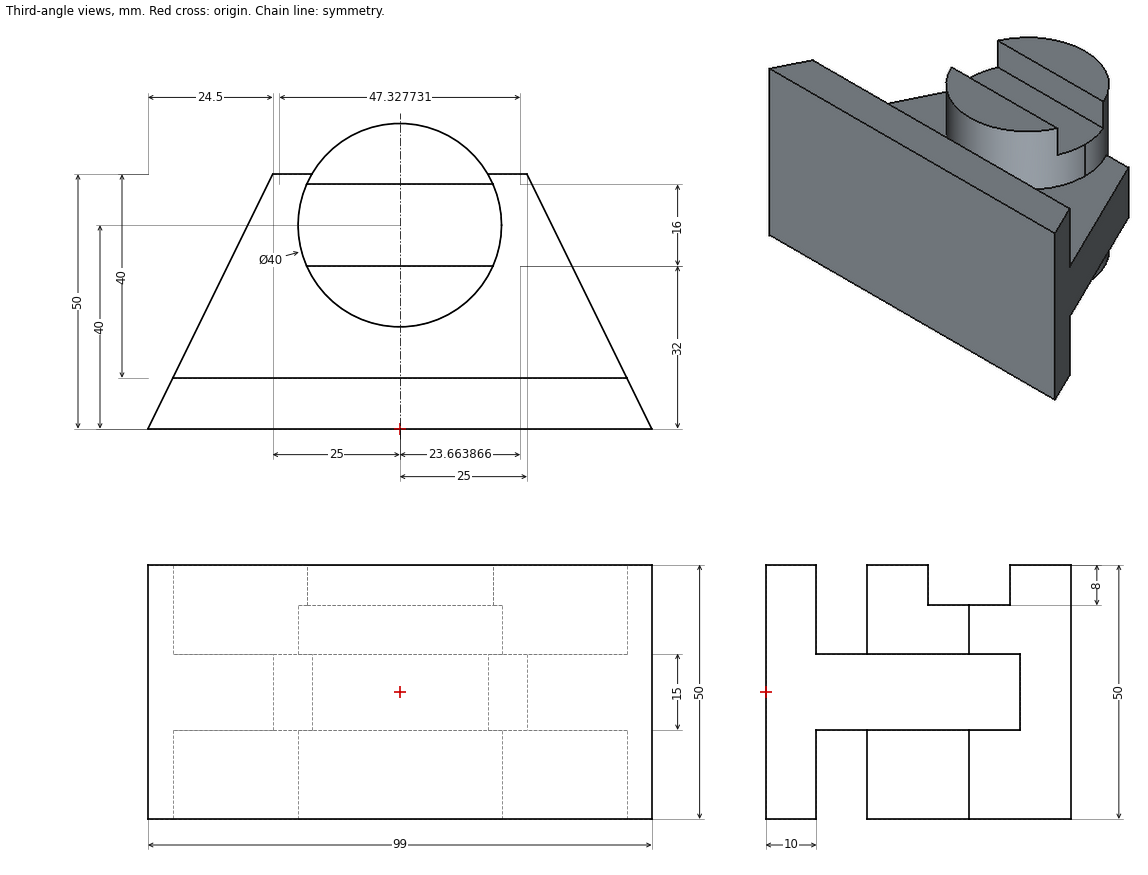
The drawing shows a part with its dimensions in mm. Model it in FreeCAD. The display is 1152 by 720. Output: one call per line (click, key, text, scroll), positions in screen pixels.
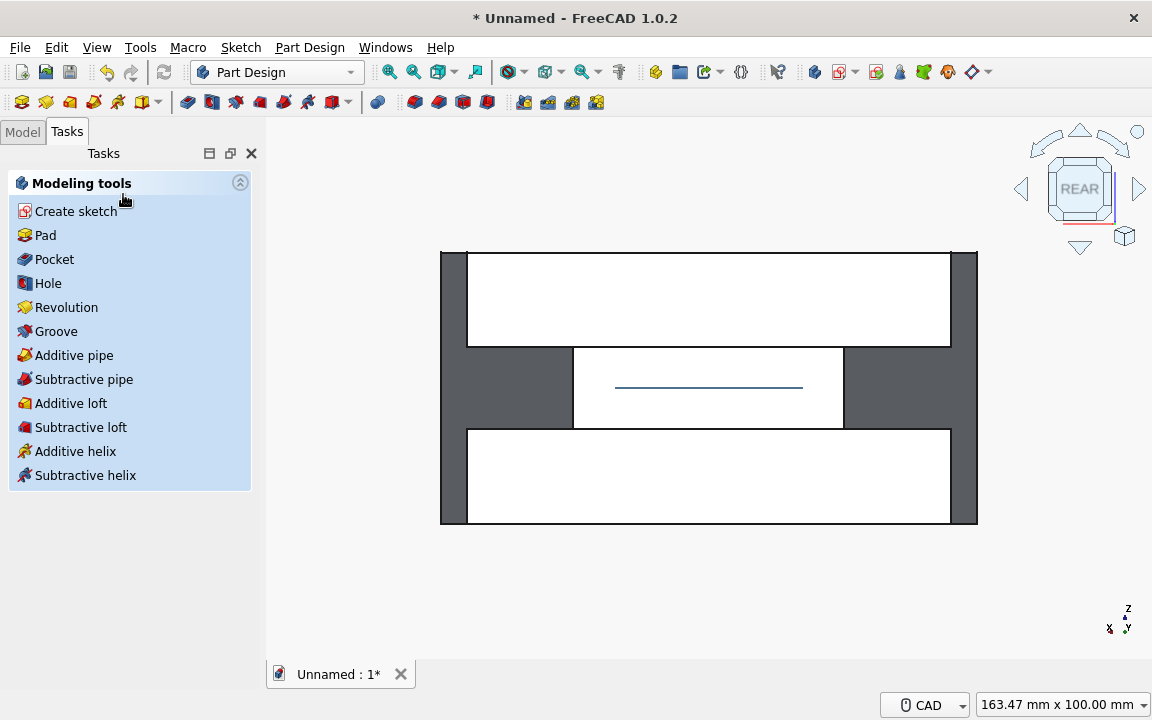
click(22, 102)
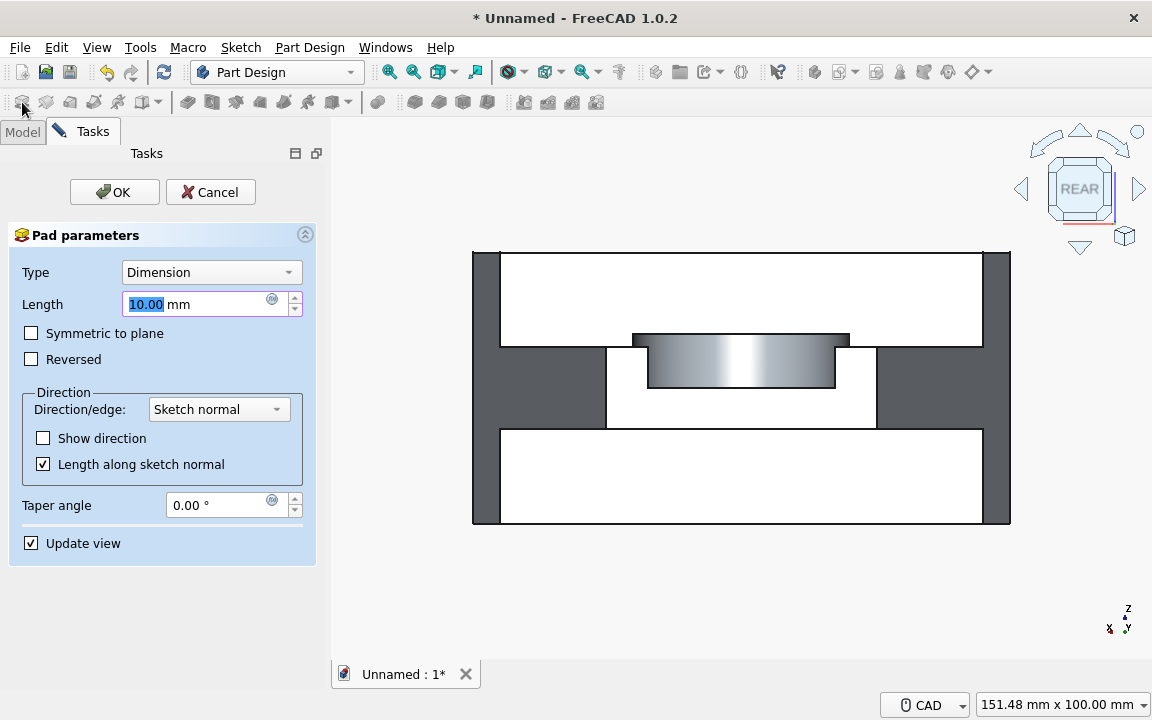
text(50)
key(Tab)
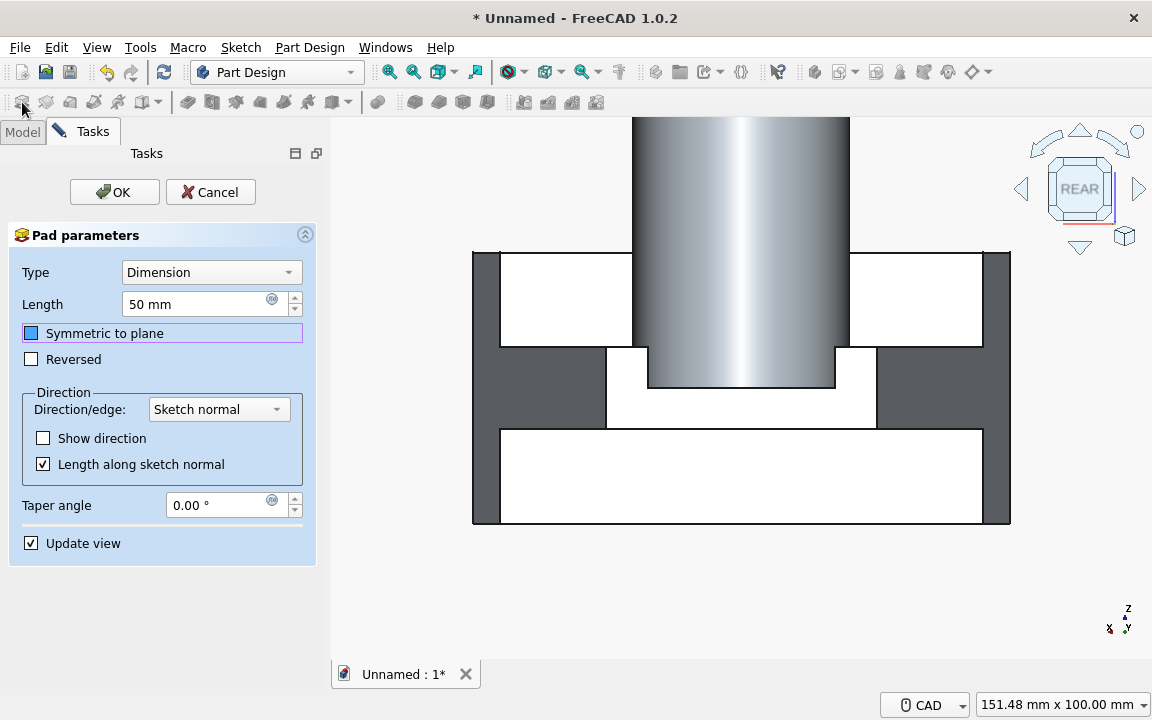
click(30, 333)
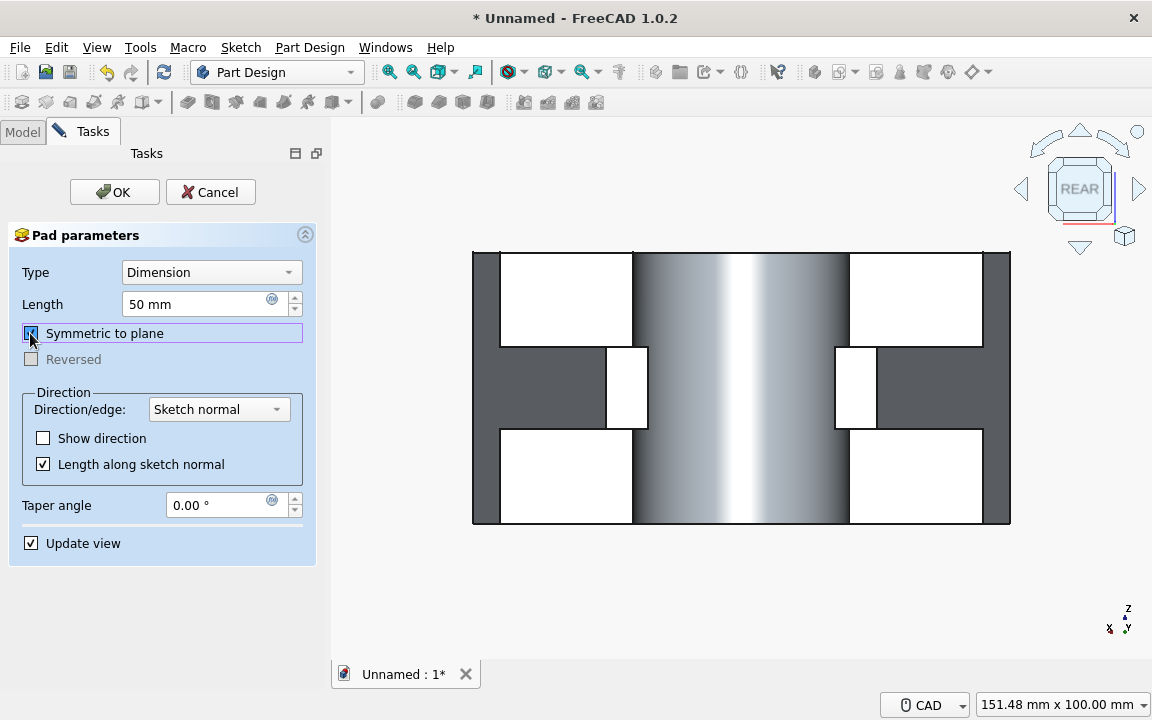
click(115, 192)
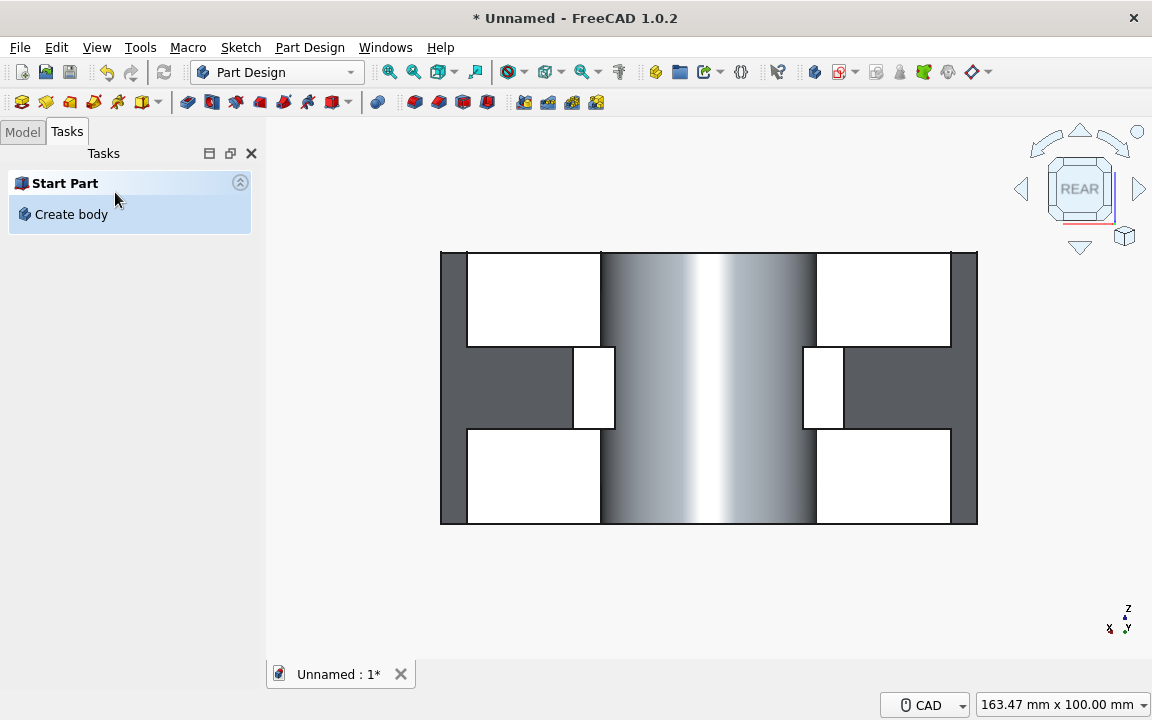
key(0)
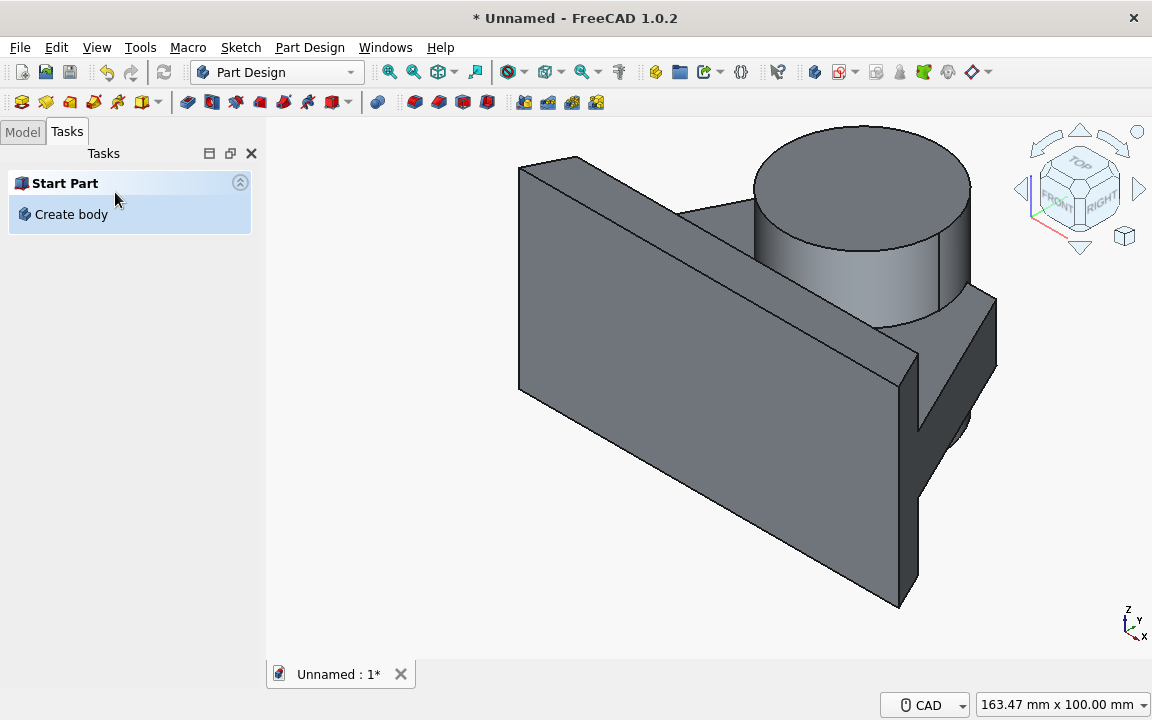
key(v)
key(f)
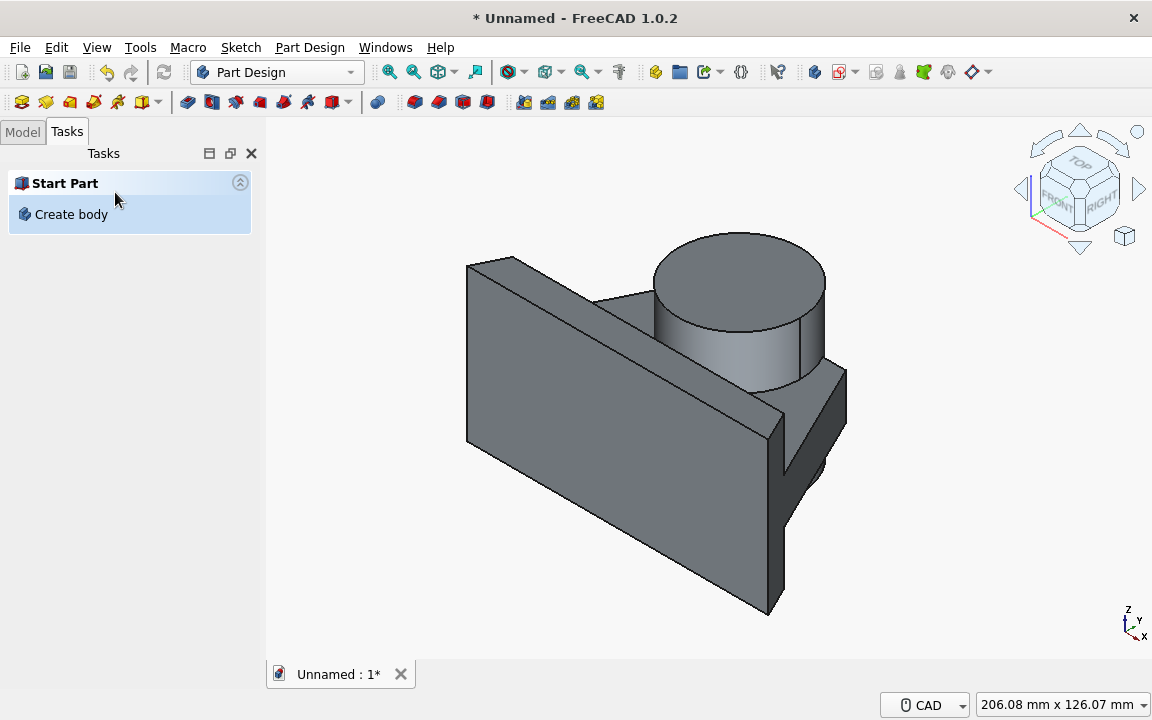
click(740, 282)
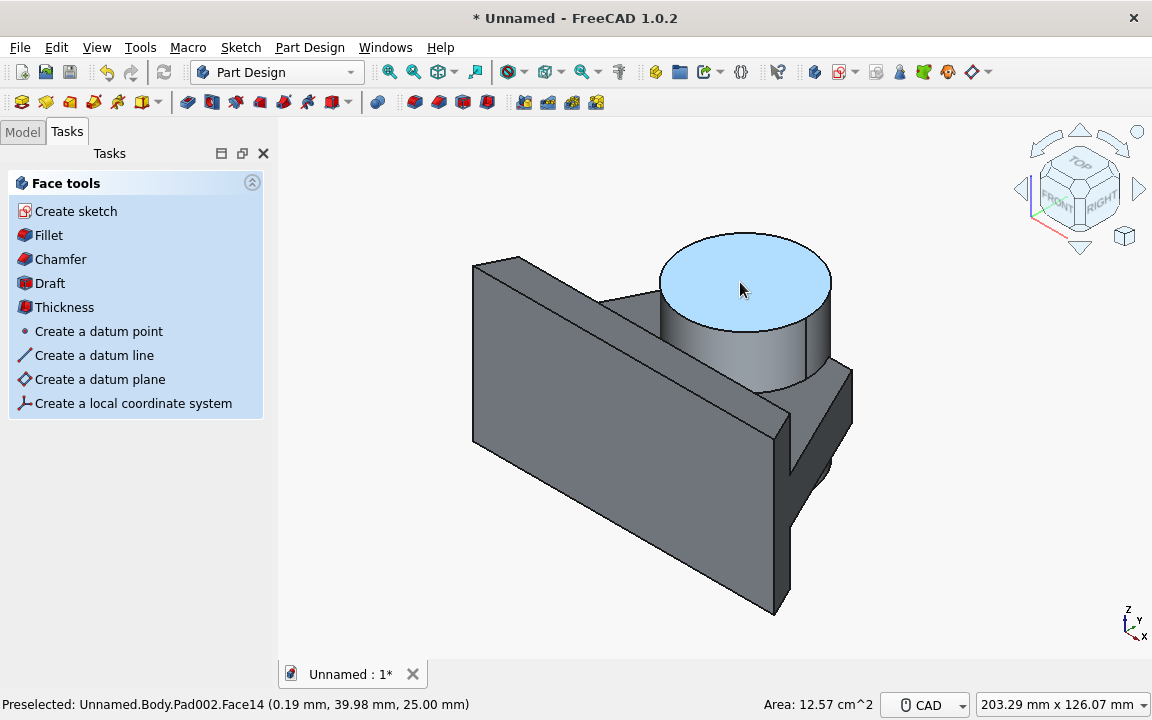
click(840, 72)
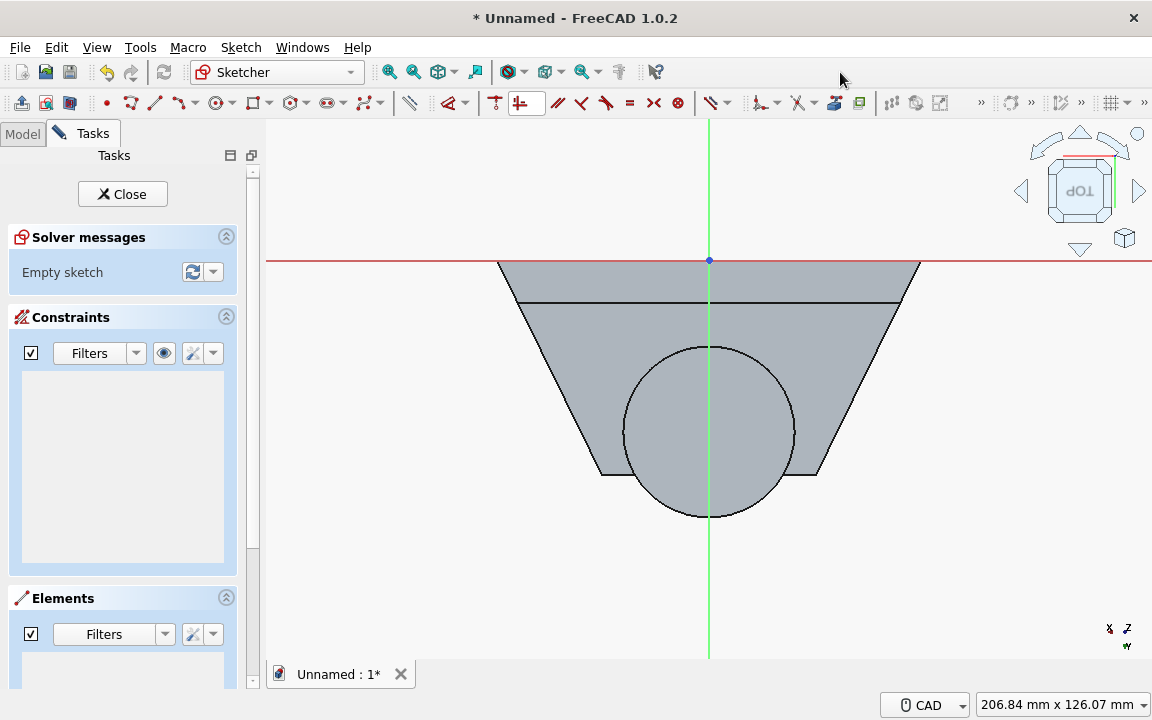
scroll(792, 332, up, 3)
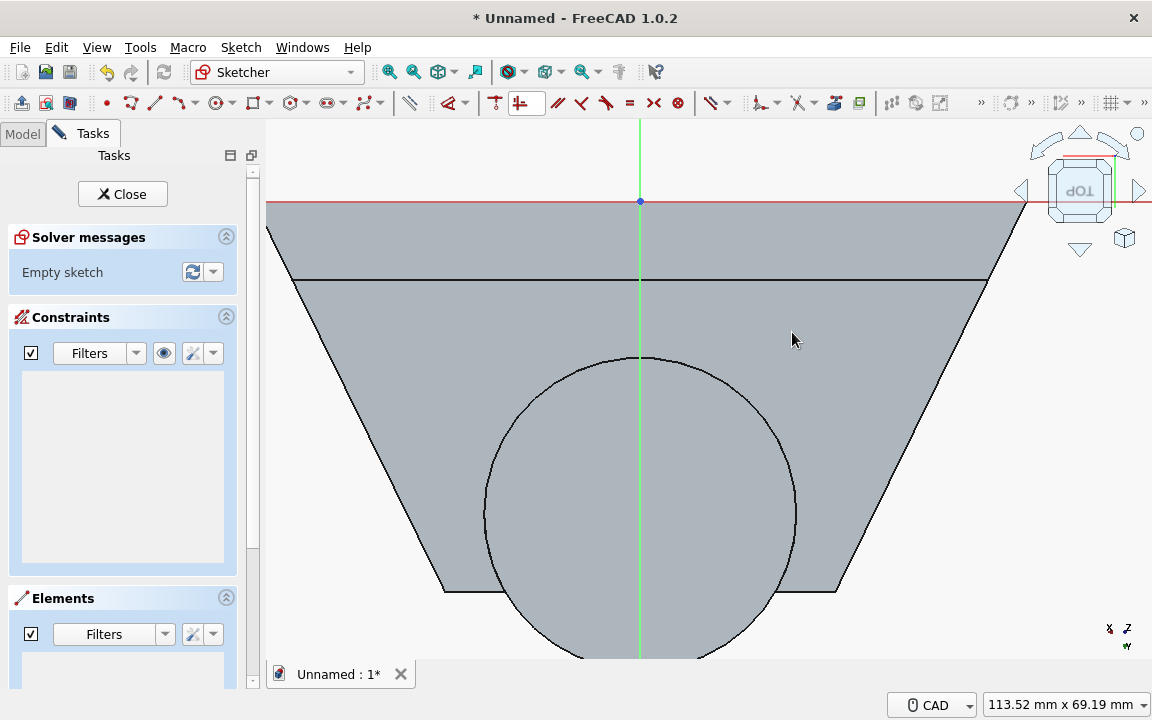
key(g)
key(r)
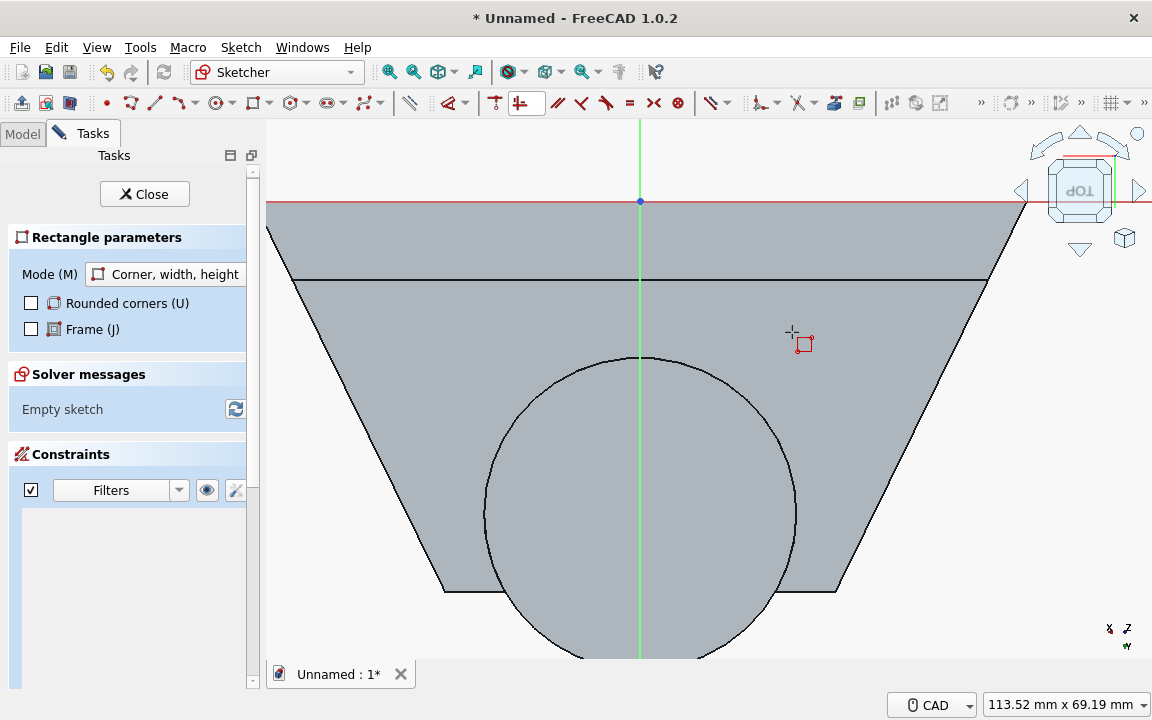
click(456, 451)
click(825, 576)
key(Escape)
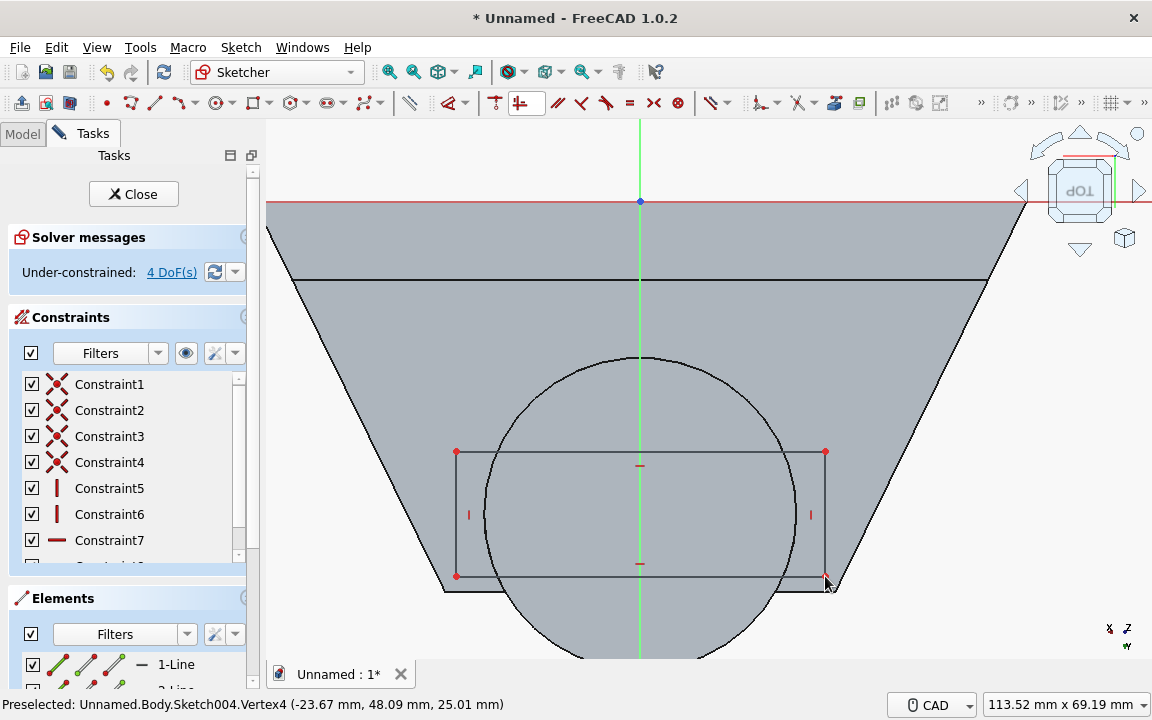
click(448, 104)